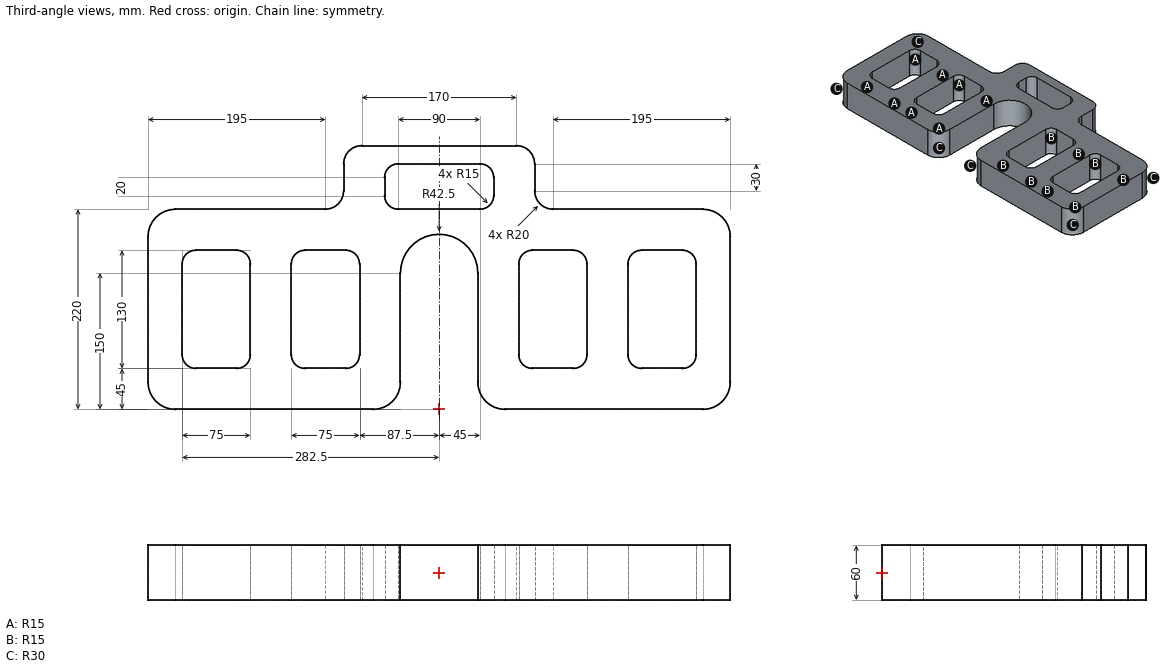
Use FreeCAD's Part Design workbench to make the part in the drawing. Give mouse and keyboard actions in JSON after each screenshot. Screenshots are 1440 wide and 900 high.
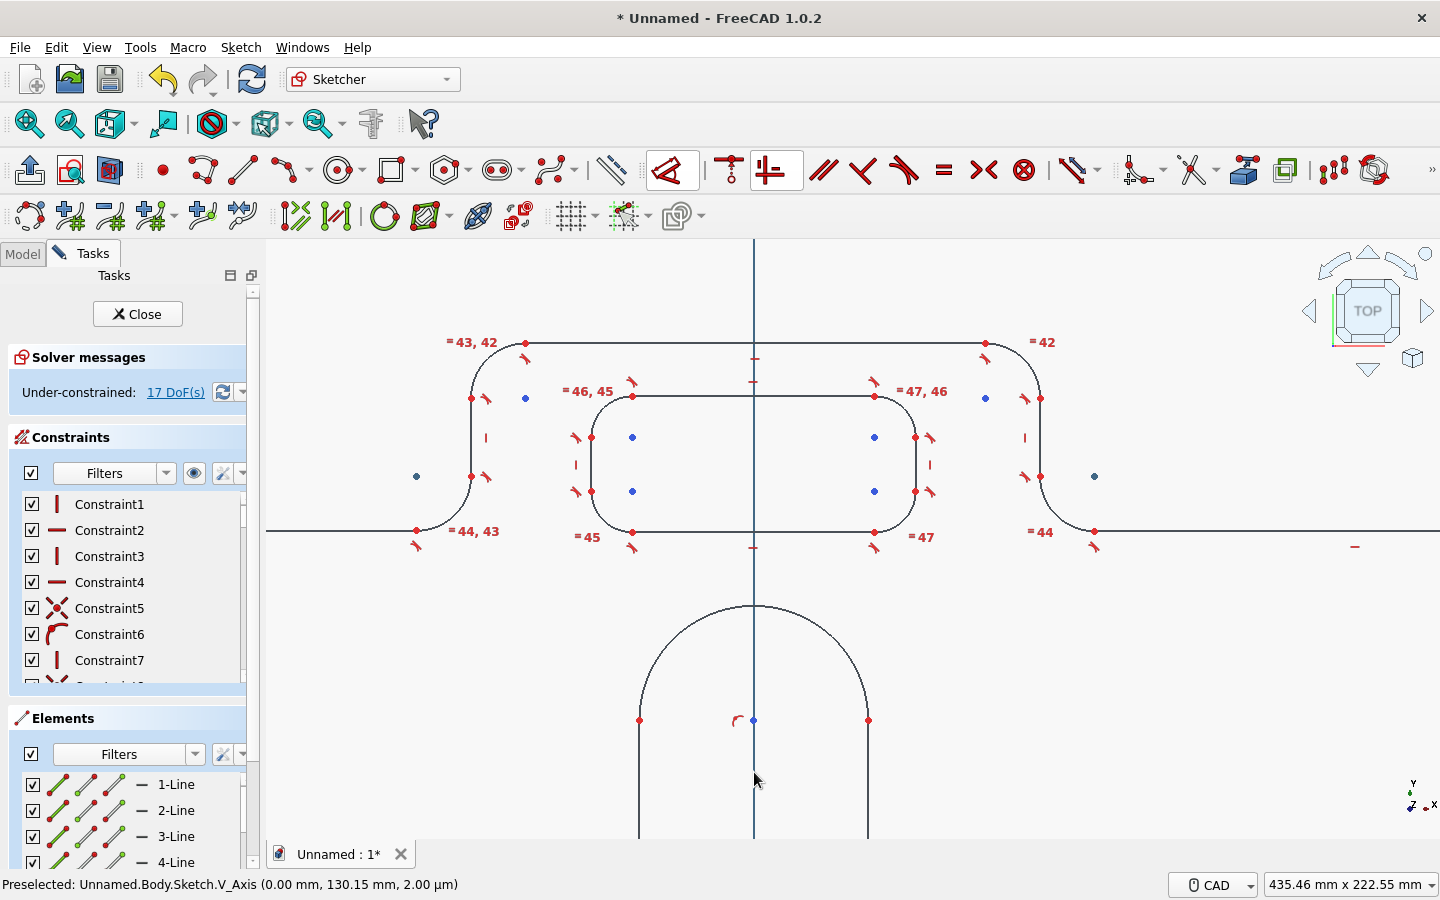
{"action": "key", "text": "s"}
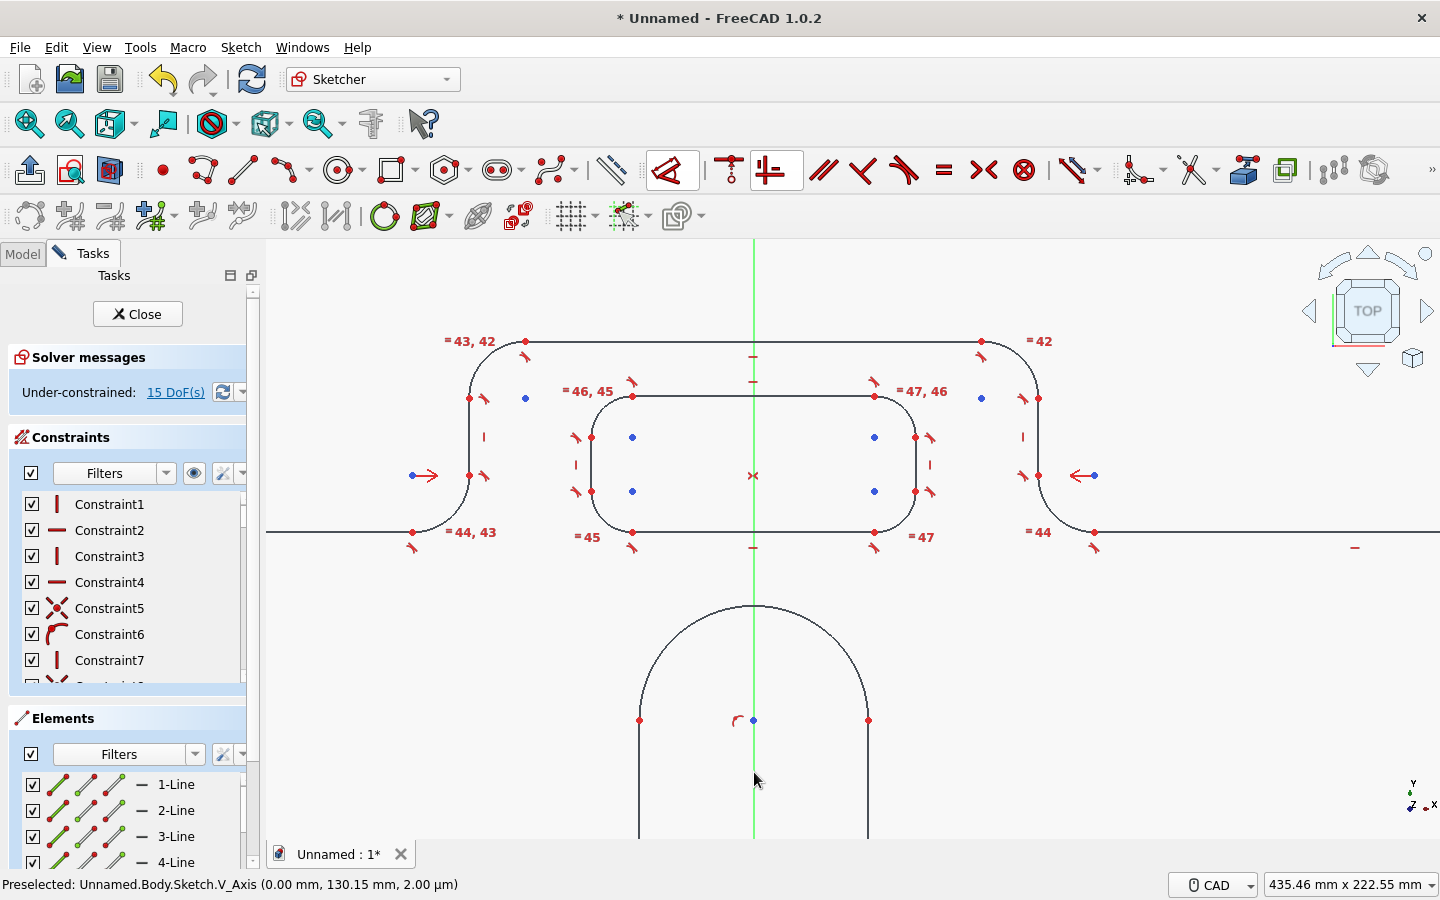
{"action": "left_click", "coordinate": [666, 170]}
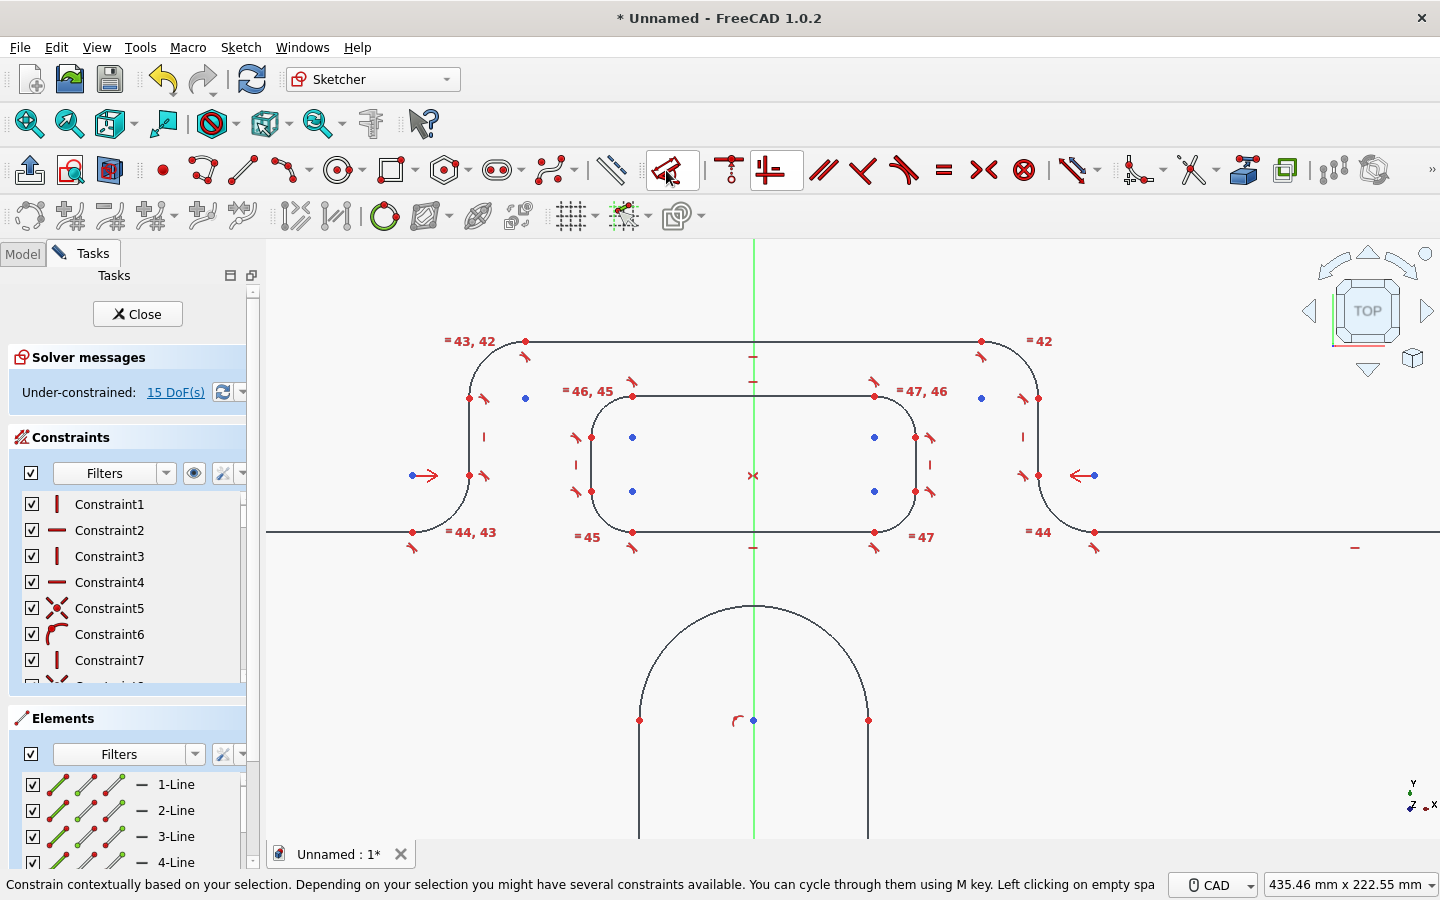
{"action": "left_click", "coordinate": [1032, 372]}
{"action": "left_click", "coordinate": [1060, 357]}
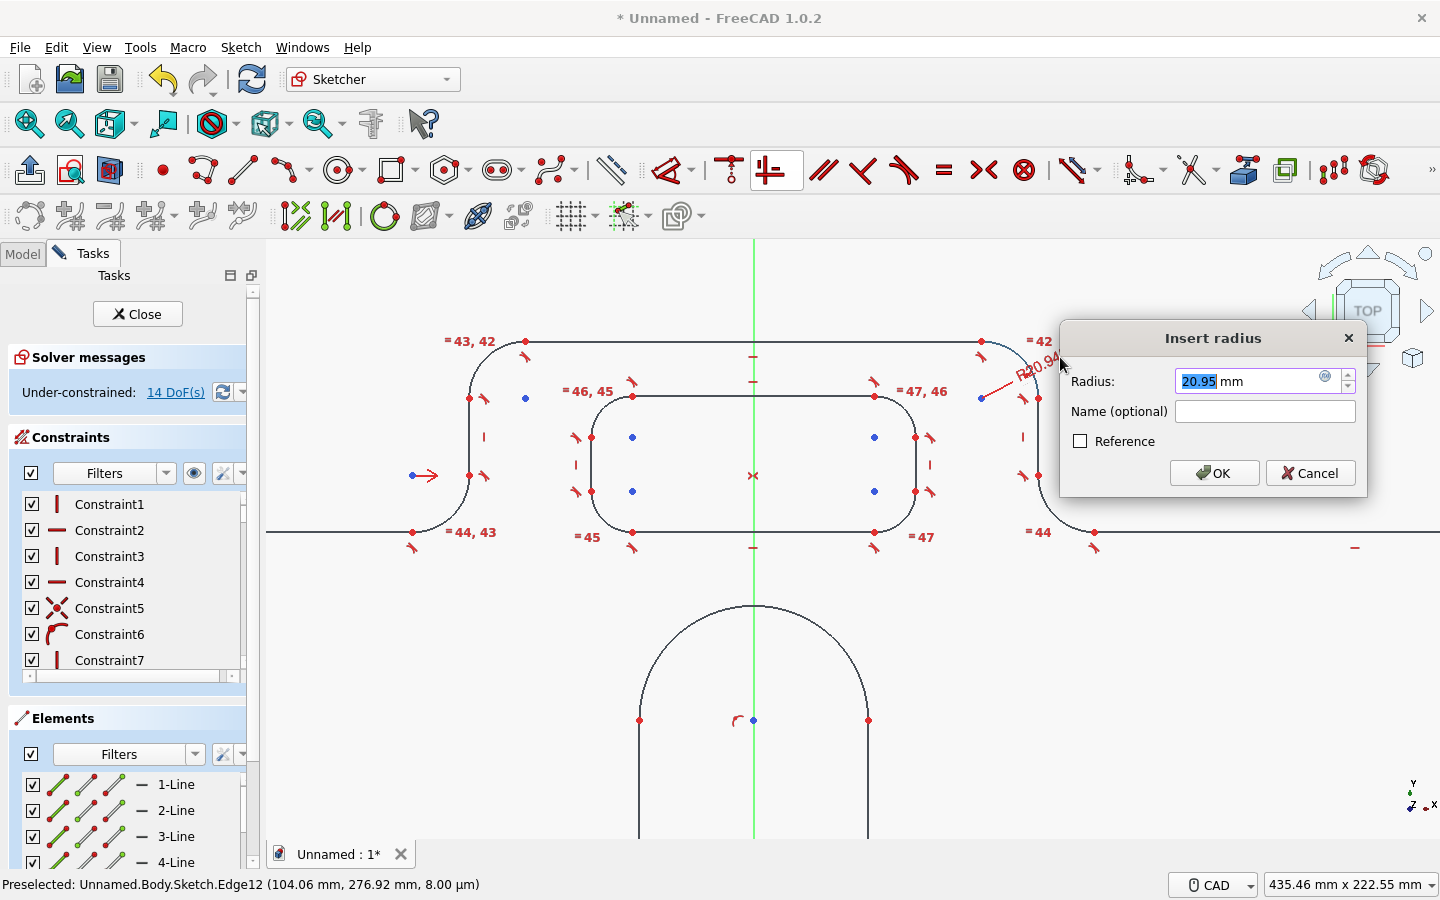
{"action": "type", "text": "20"}
{"action": "key", "text": "Return"}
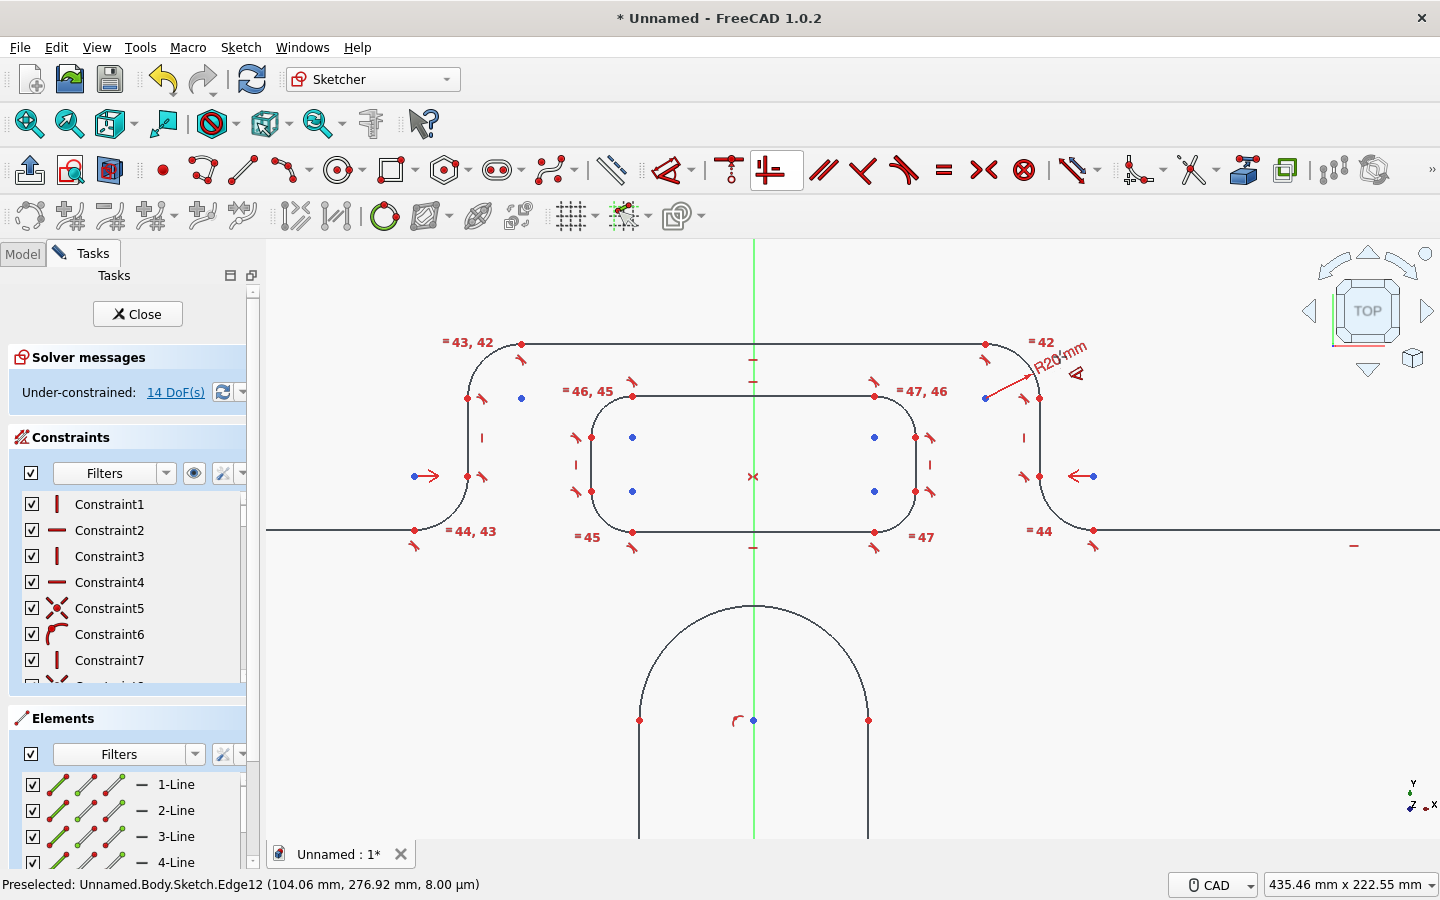
{"action": "left_click", "coordinate": [821, 628]}
{"action": "left_click", "coordinate": [840, 602]}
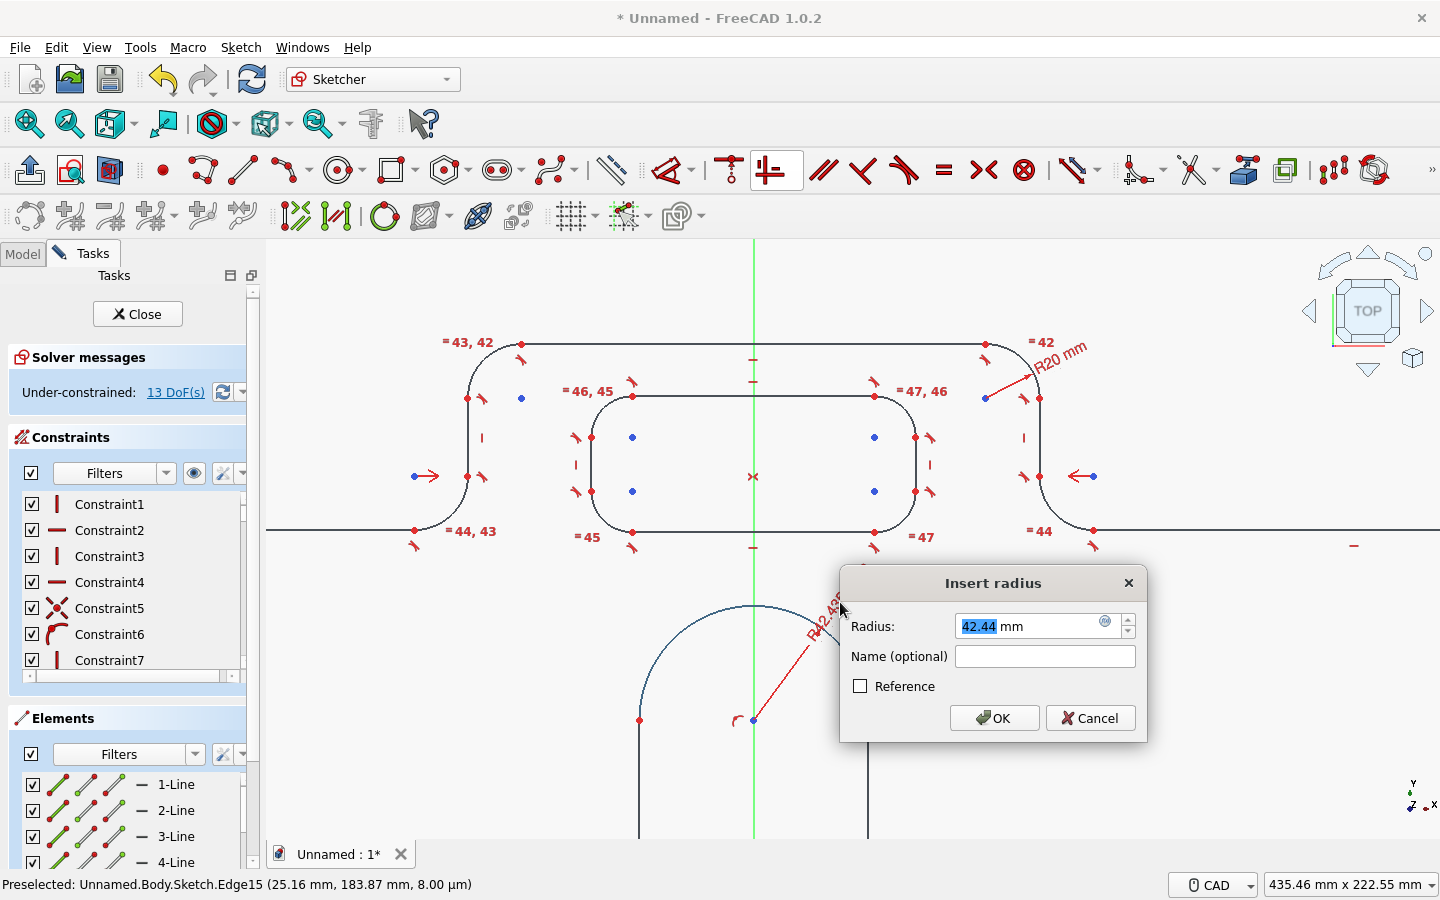
{"action": "type", "text": "42.5"}
{"action": "key", "text": "Return"}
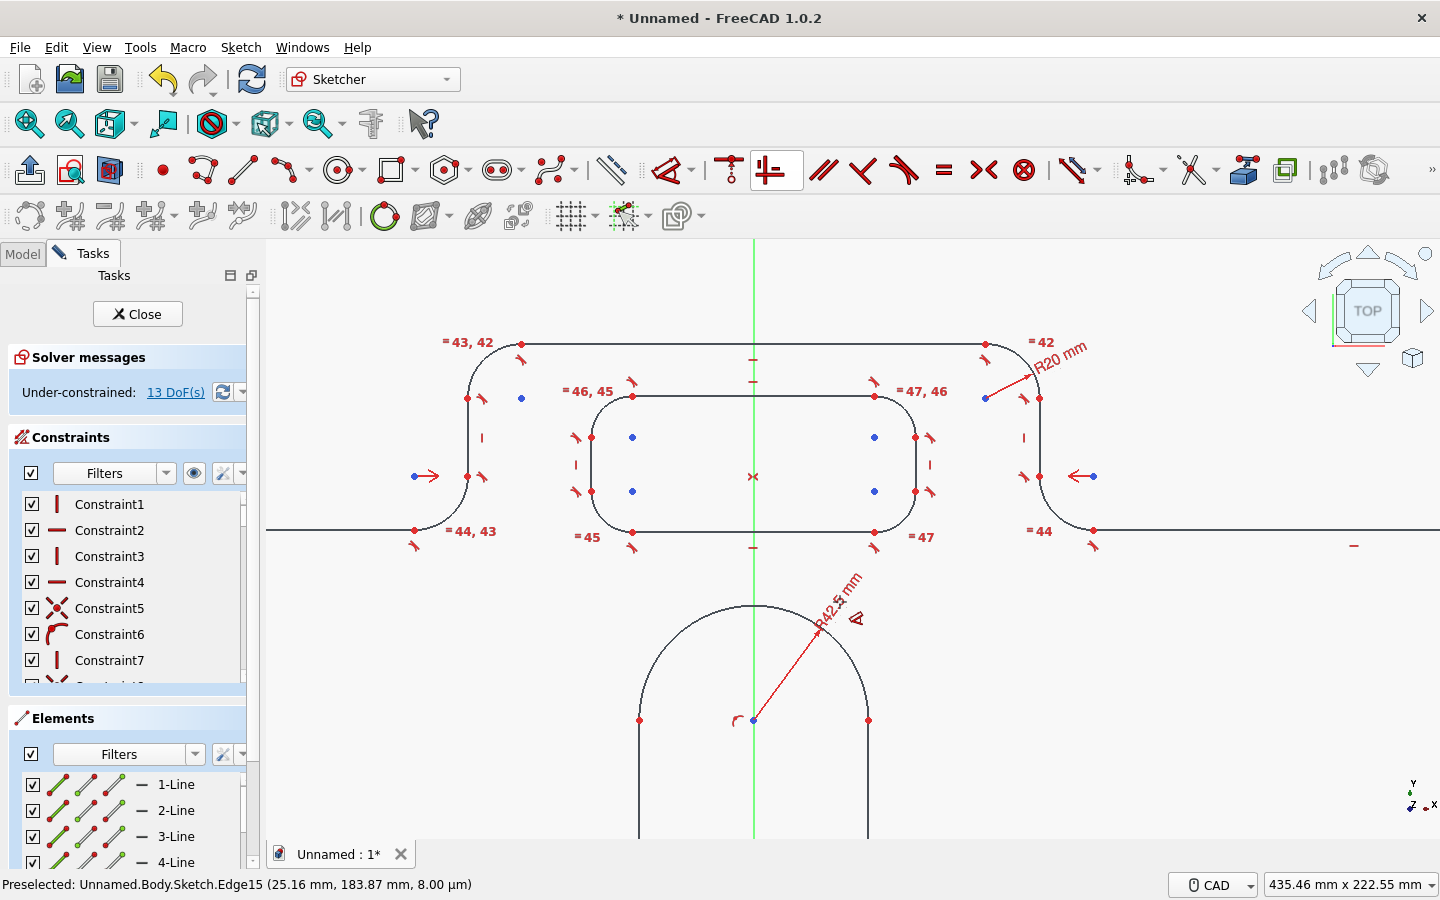
{"action": "left_click", "coordinate": [596, 510]}
{"action": "left_click", "coordinate": [568, 525]}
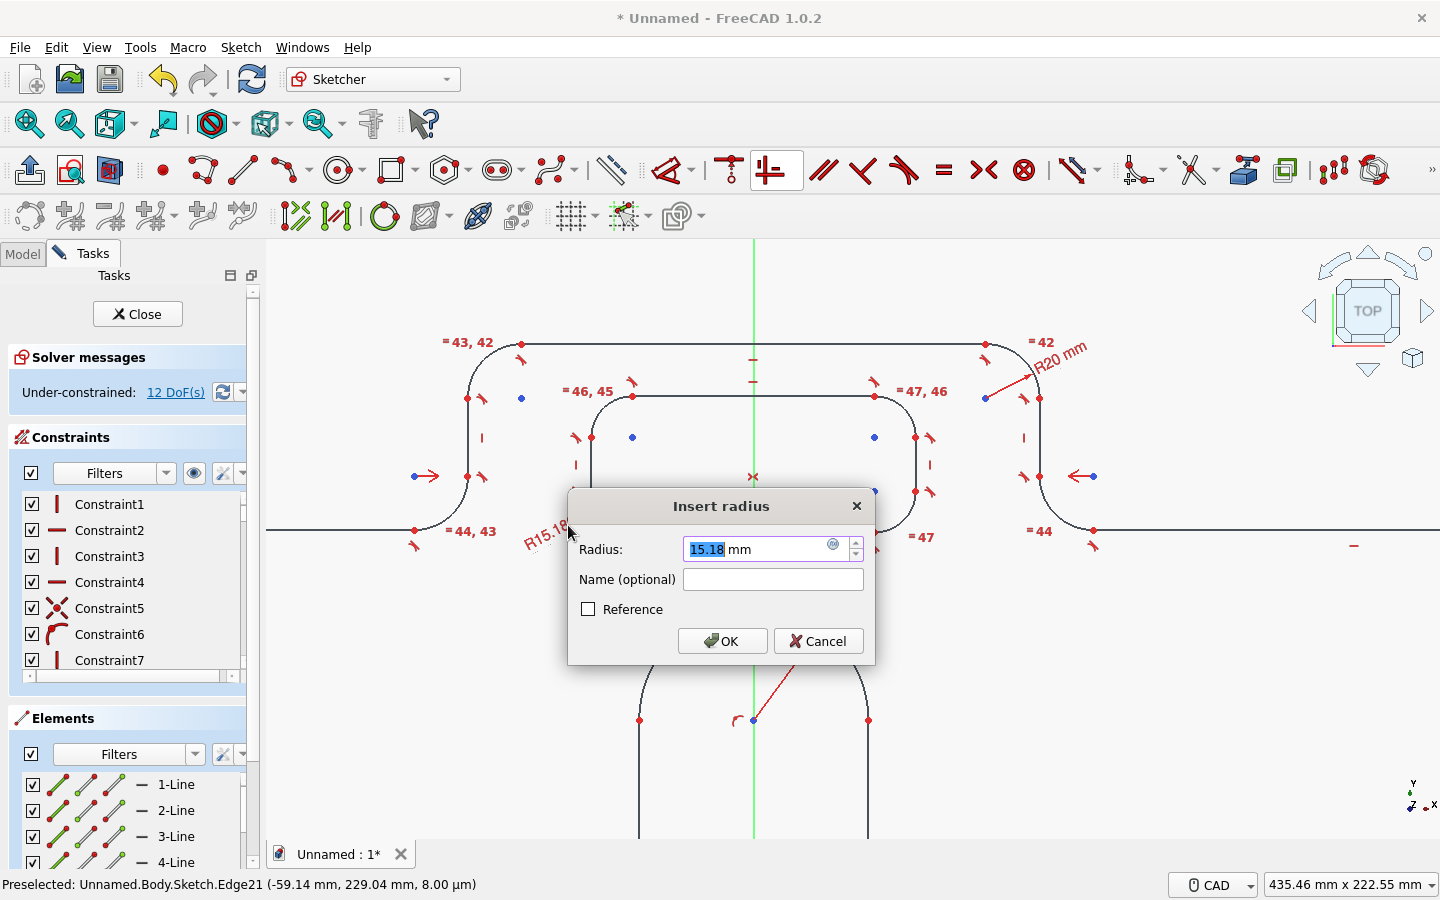
{"action": "type", "text": "15"}
{"action": "key", "text": "Return"}